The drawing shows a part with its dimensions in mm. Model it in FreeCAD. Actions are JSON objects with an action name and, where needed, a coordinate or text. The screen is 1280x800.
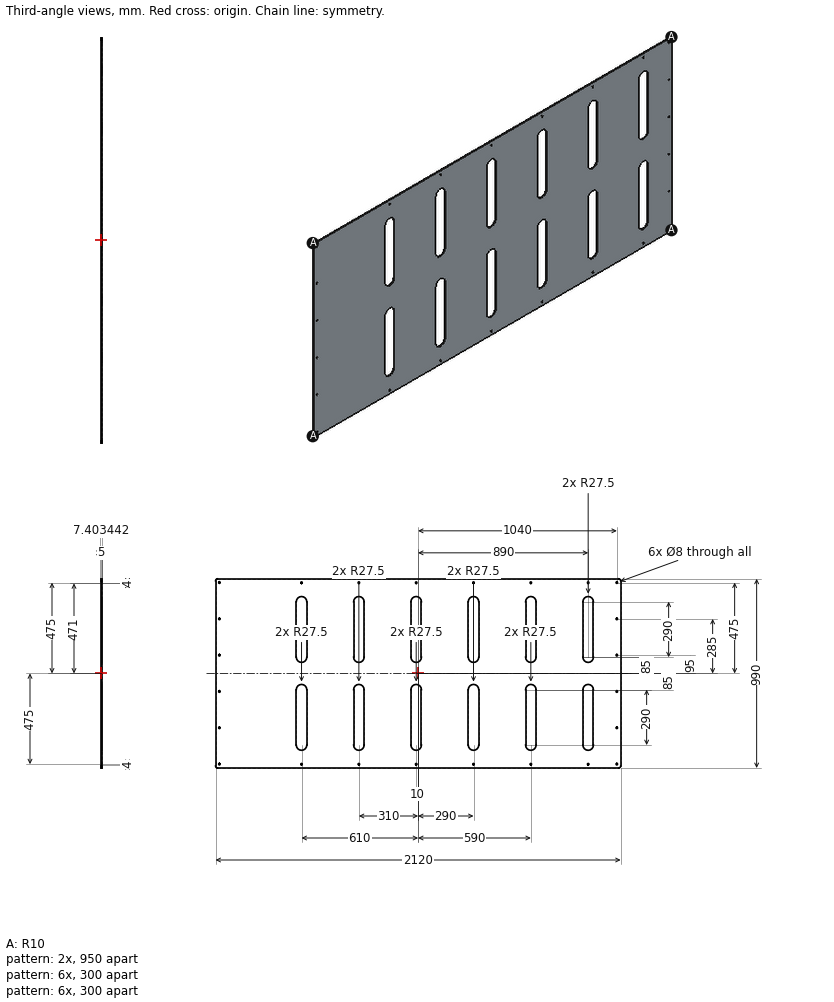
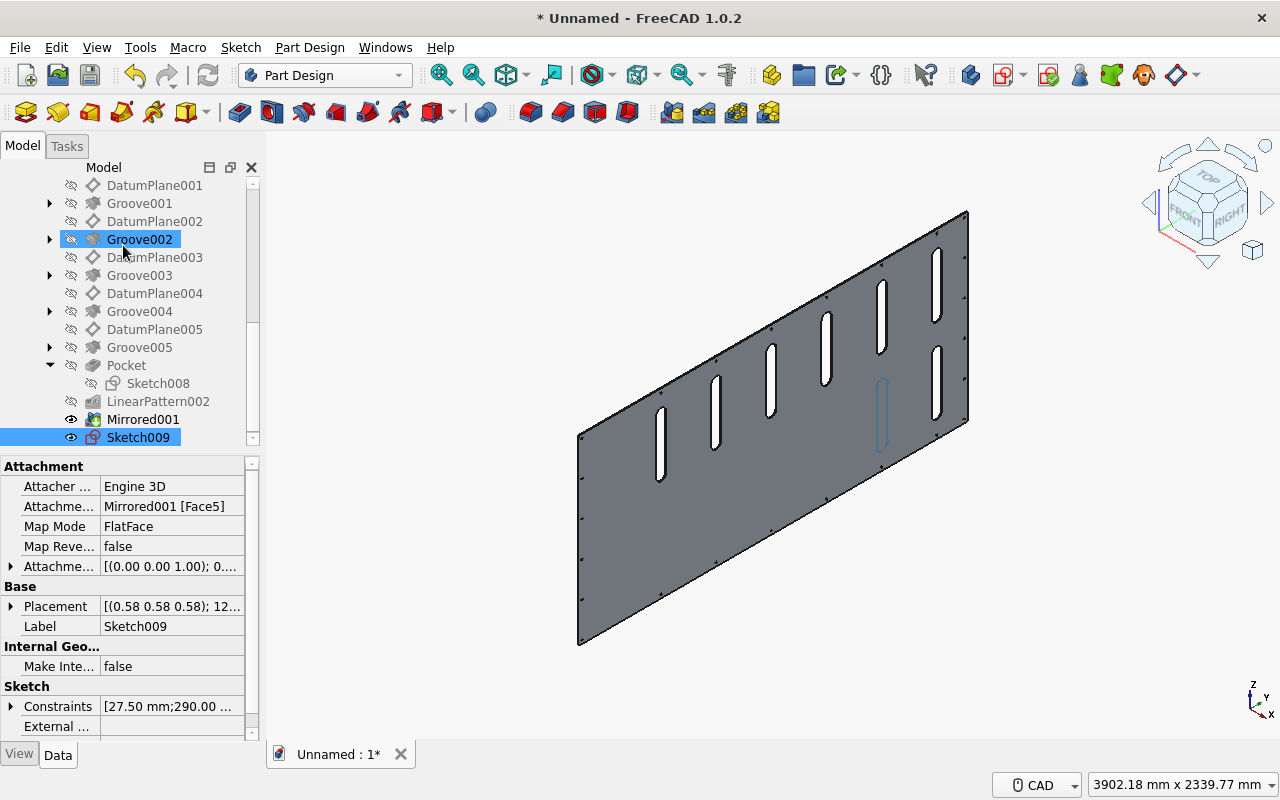
{"action": "left_click", "coordinate": [240, 112]}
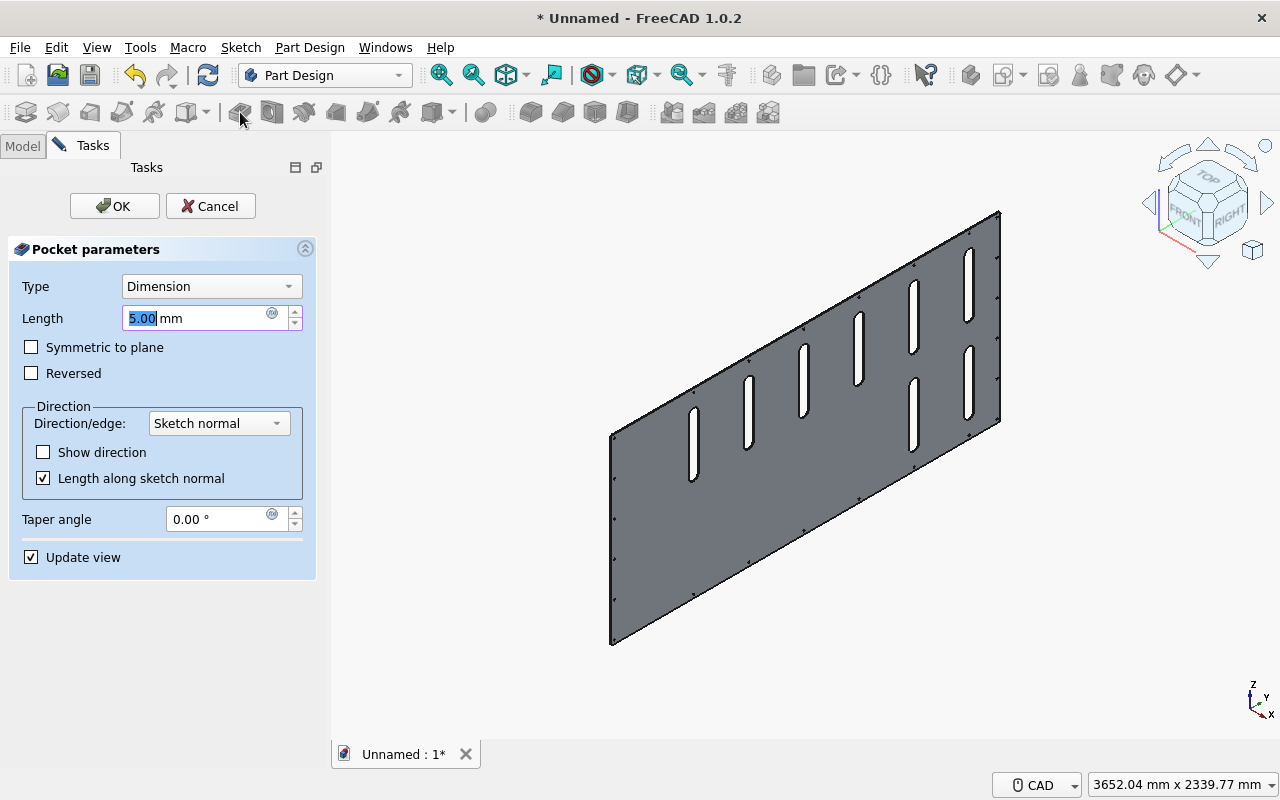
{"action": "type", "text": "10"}
{"action": "key", "text": "Tab"}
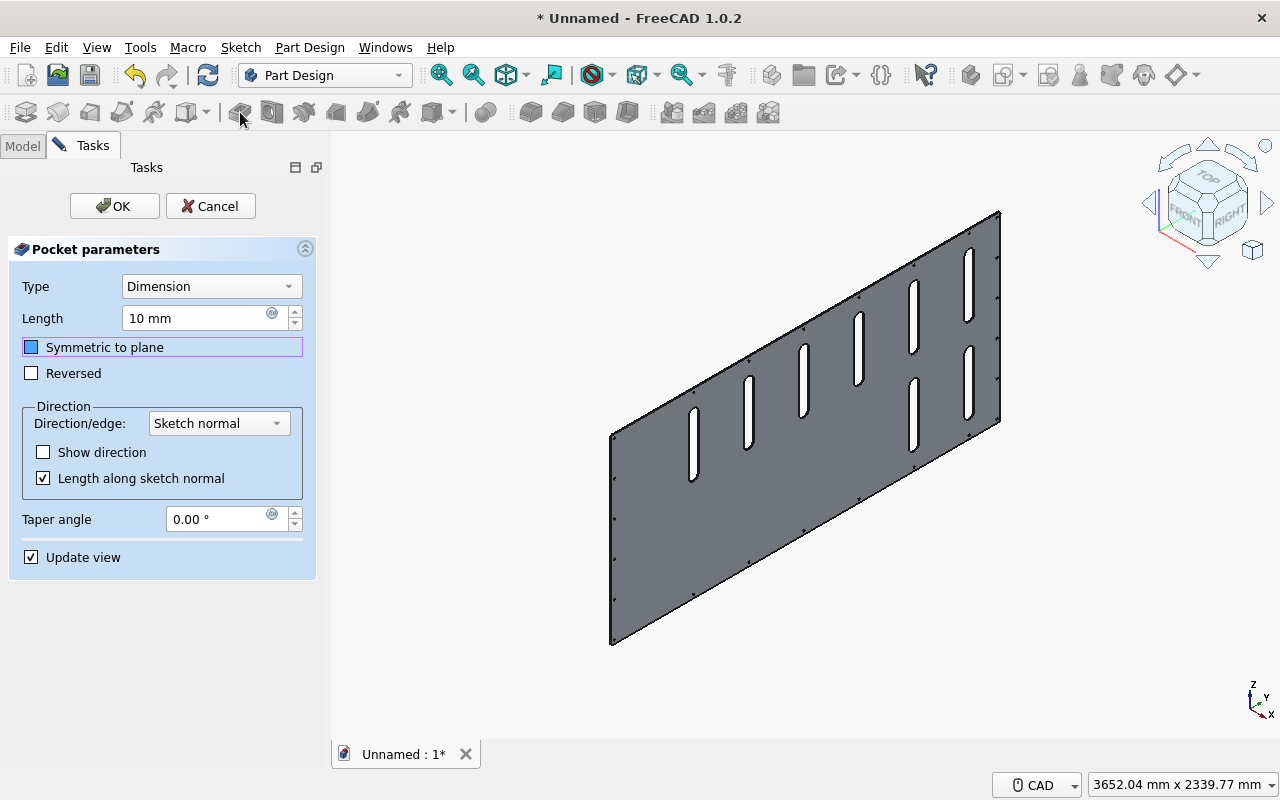
{"action": "left_click", "coordinate": [115, 206]}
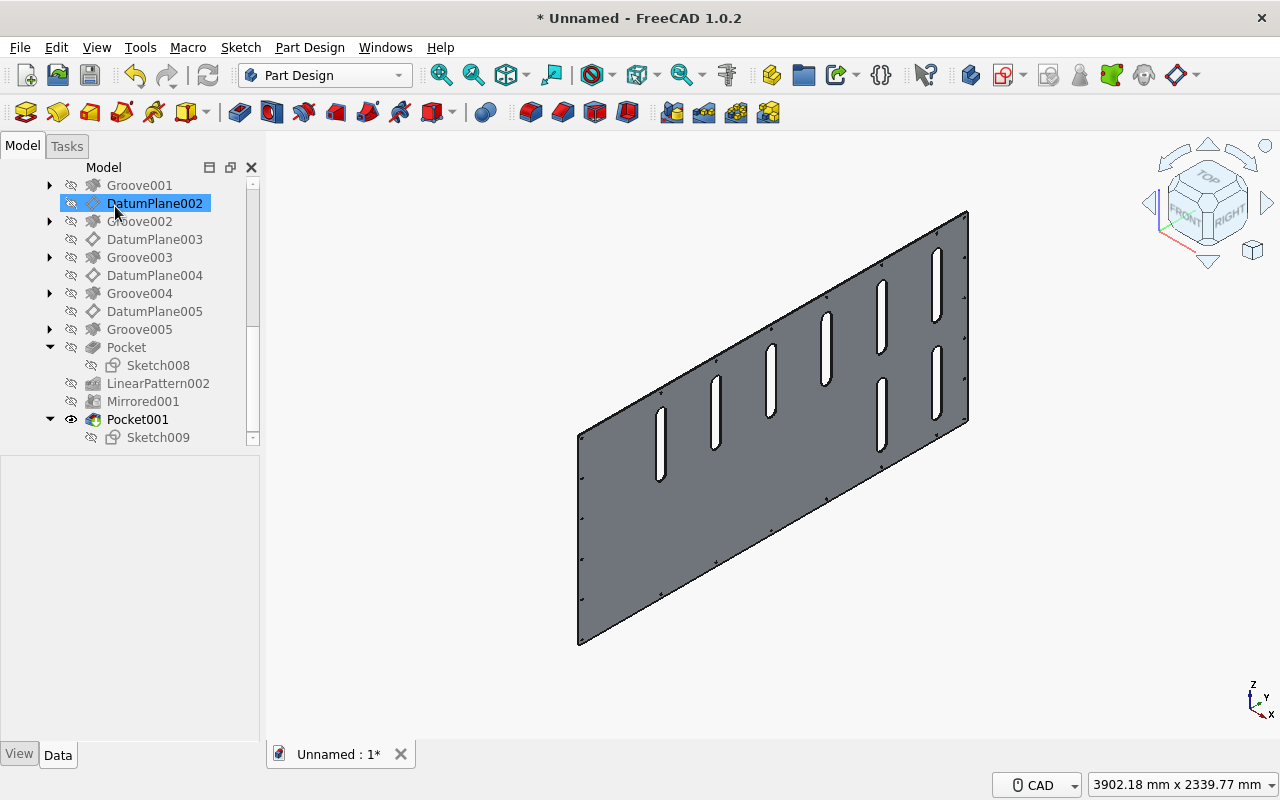
{"action": "left_click", "coordinate": [829, 426]}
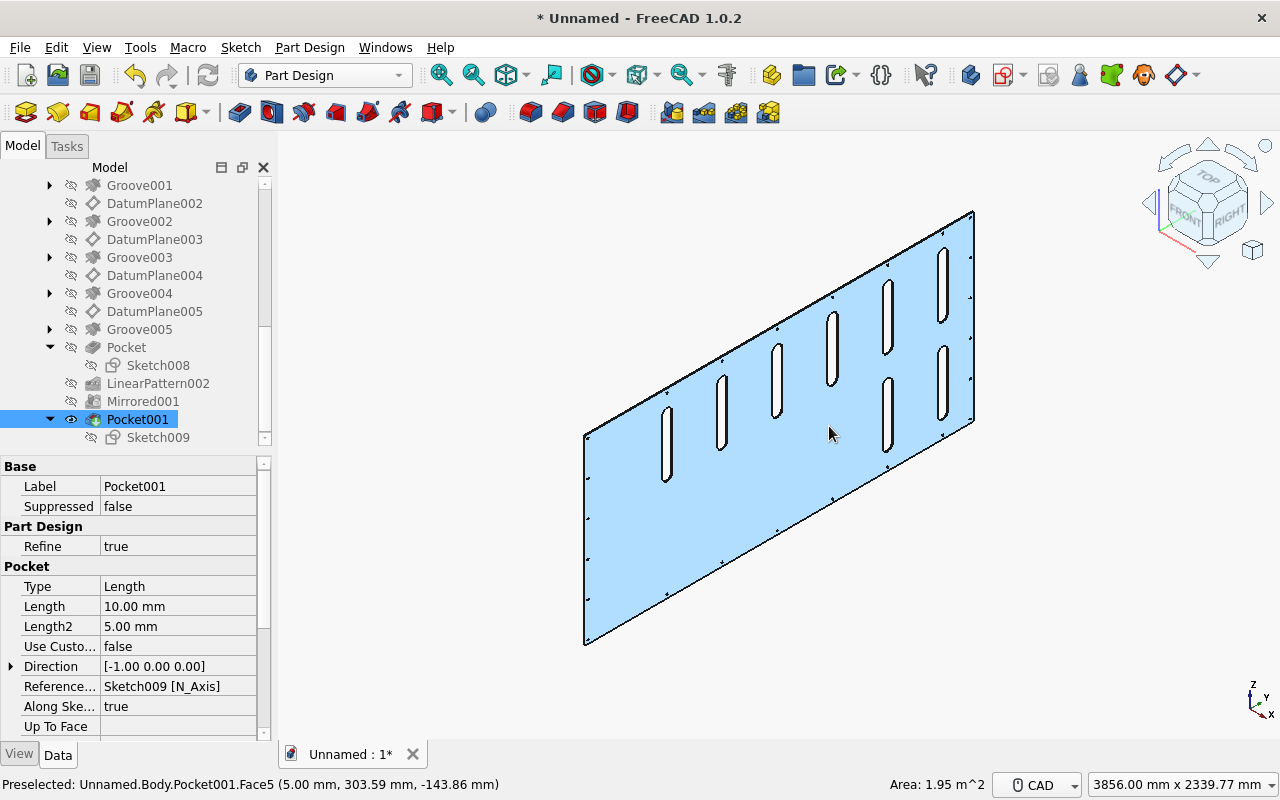
{"action": "left_click", "coordinate": [1004, 76]}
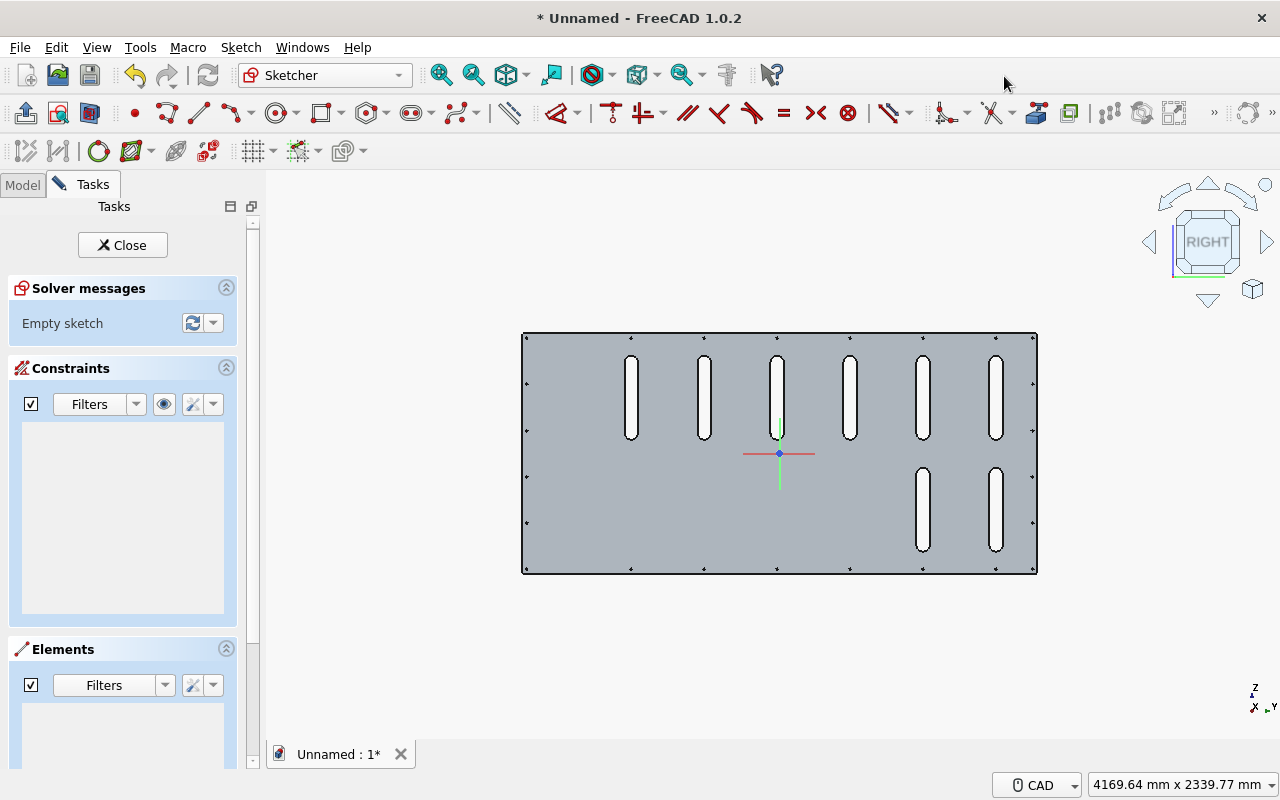
{"action": "scroll", "coordinate": [855, 518], "scroll_direction": "up", "scroll_amount": 7}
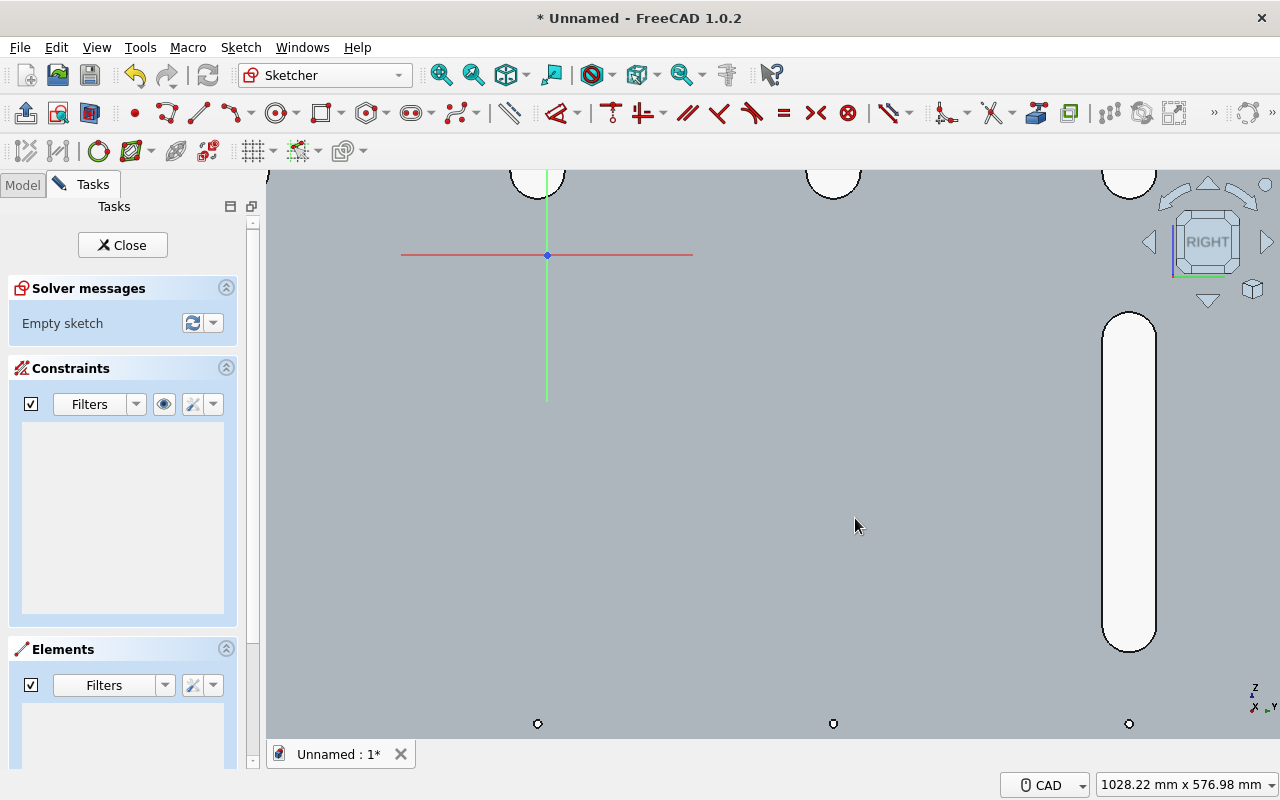
{"action": "left_click", "coordinate": [412, 114]}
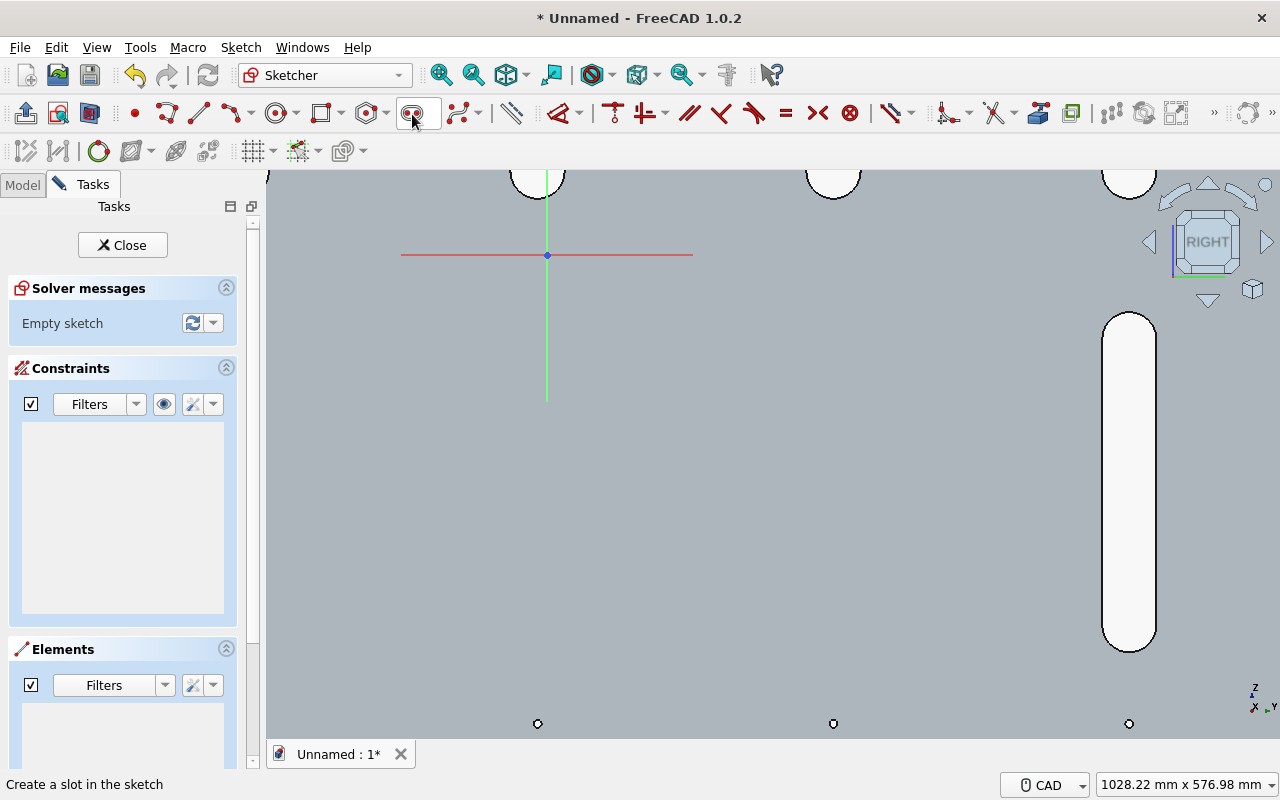
{"action": "left_click", "coordinate": [833, 625]}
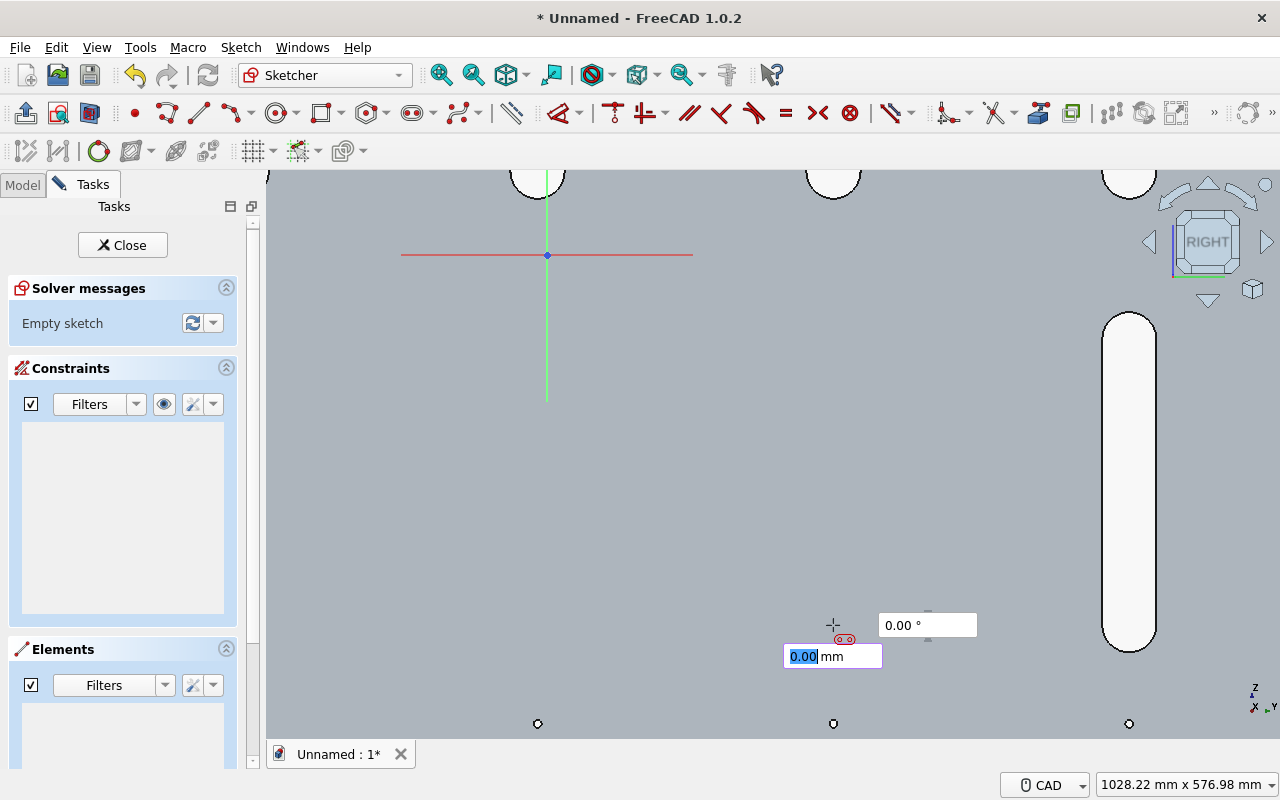
{"action": "left_click", "coordinate": [833, 339]}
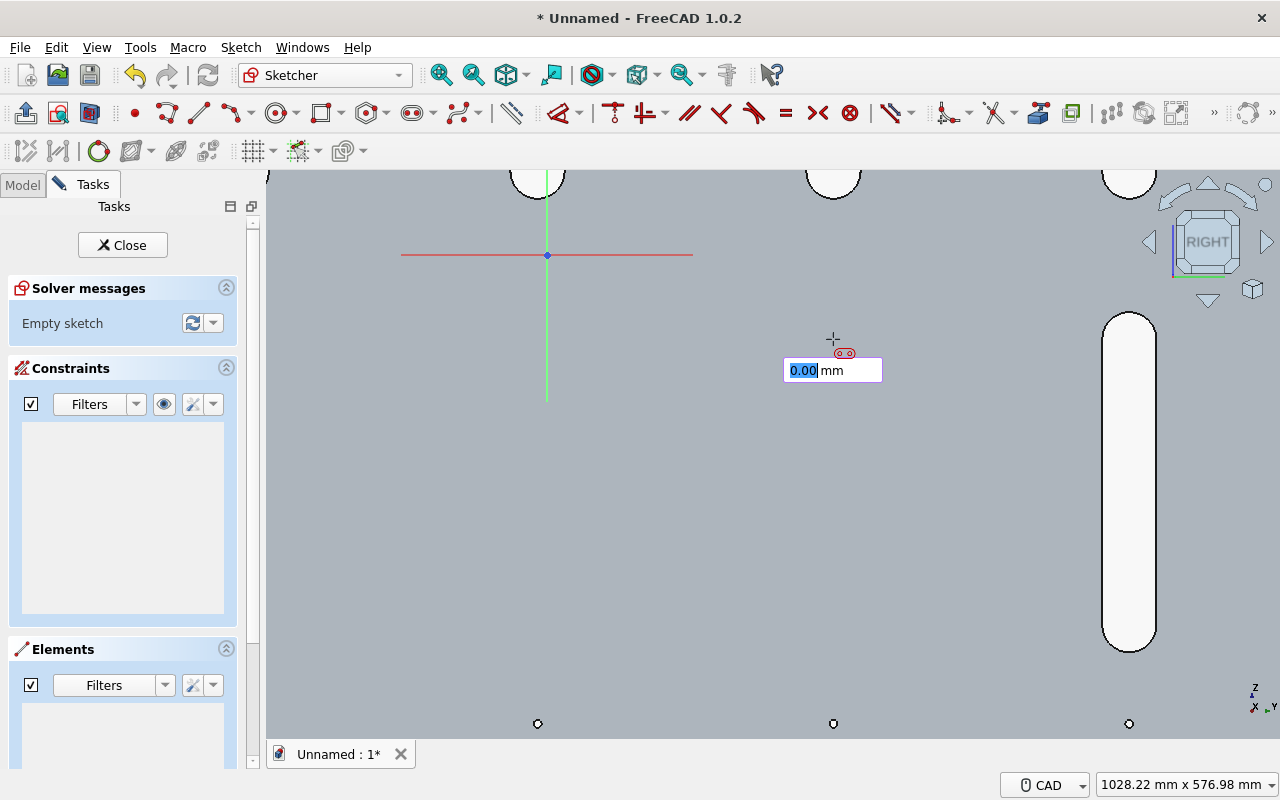
{"action": "left_click", "coordinate": [861, 482]}
{"action": "key", "text": "Escape"}